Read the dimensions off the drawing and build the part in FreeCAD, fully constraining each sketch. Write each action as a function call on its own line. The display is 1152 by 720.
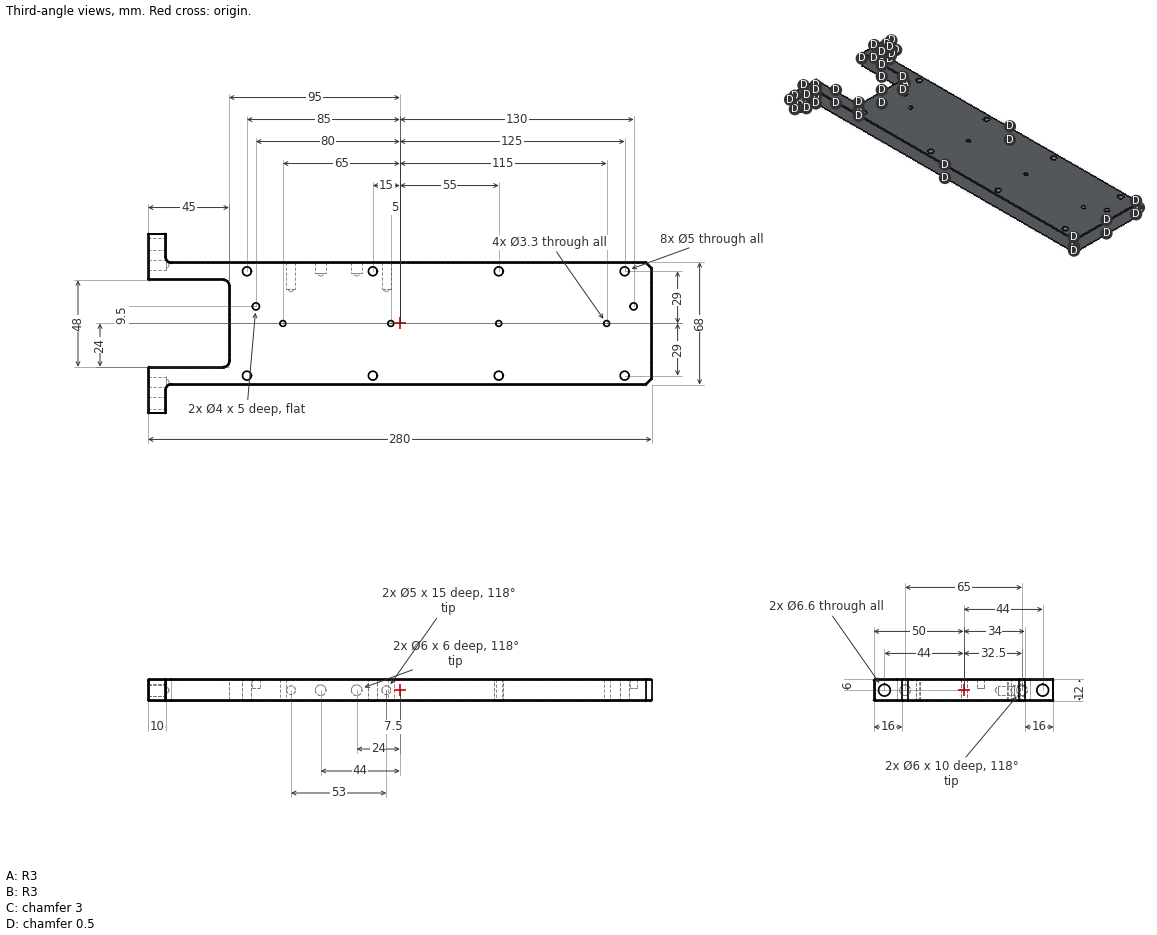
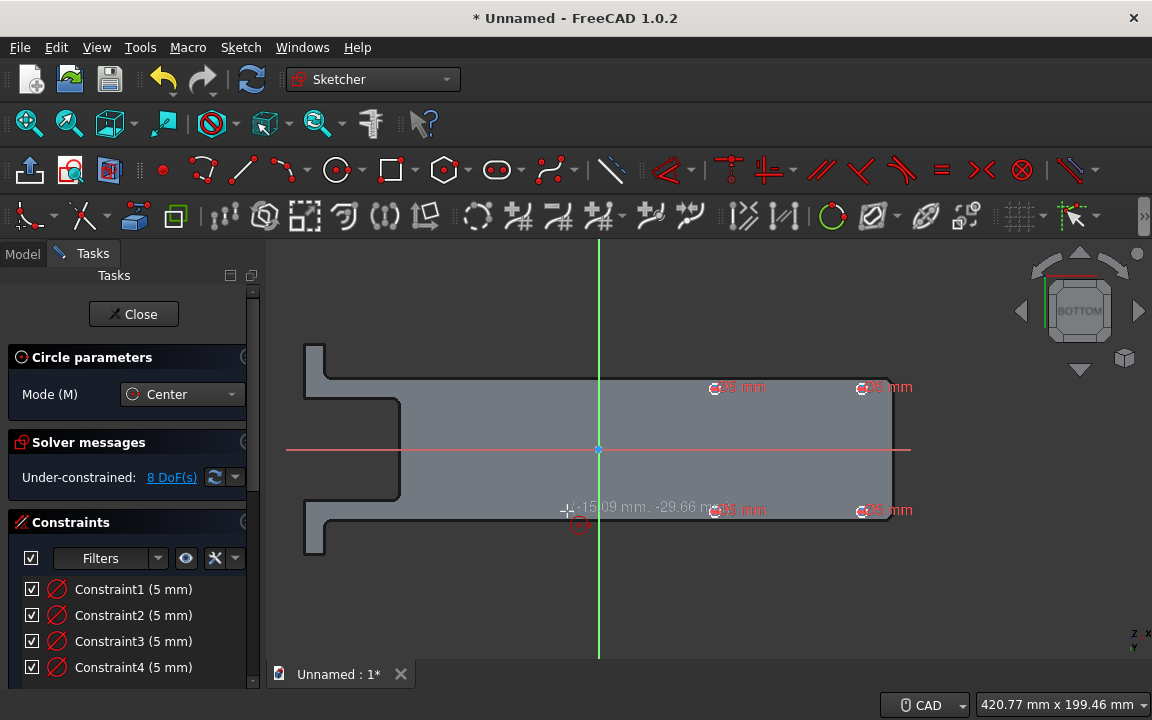
click(567, 511)
move(571, 507)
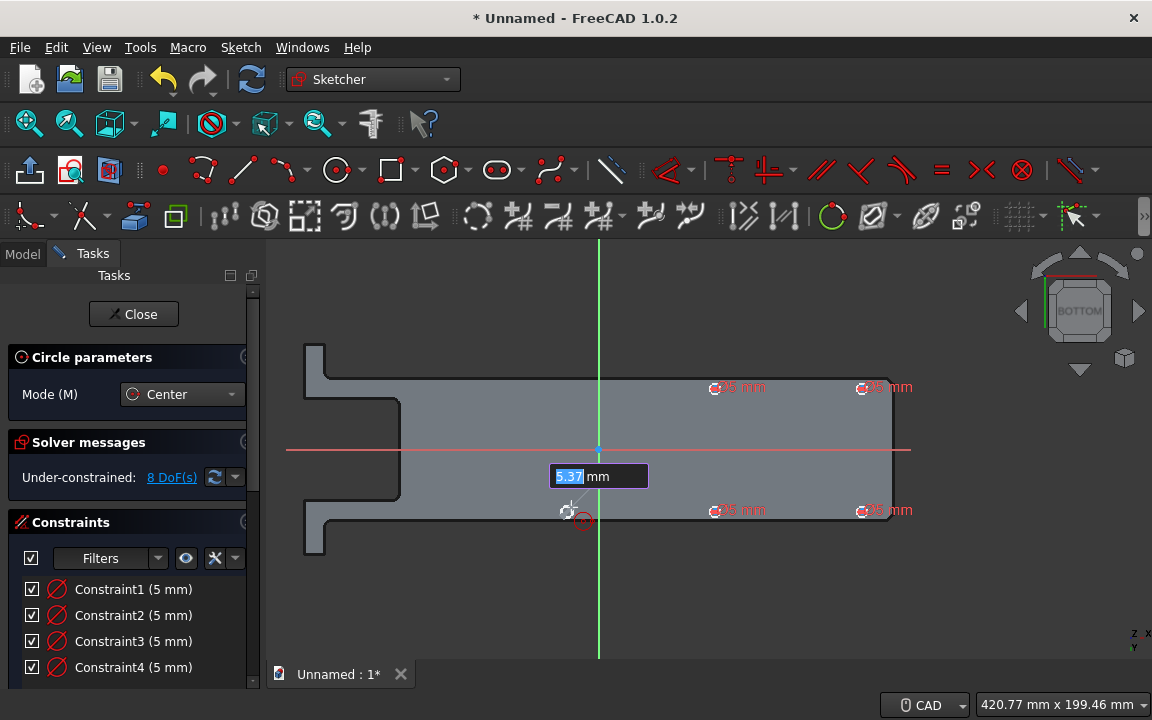
text(5)
key(Return)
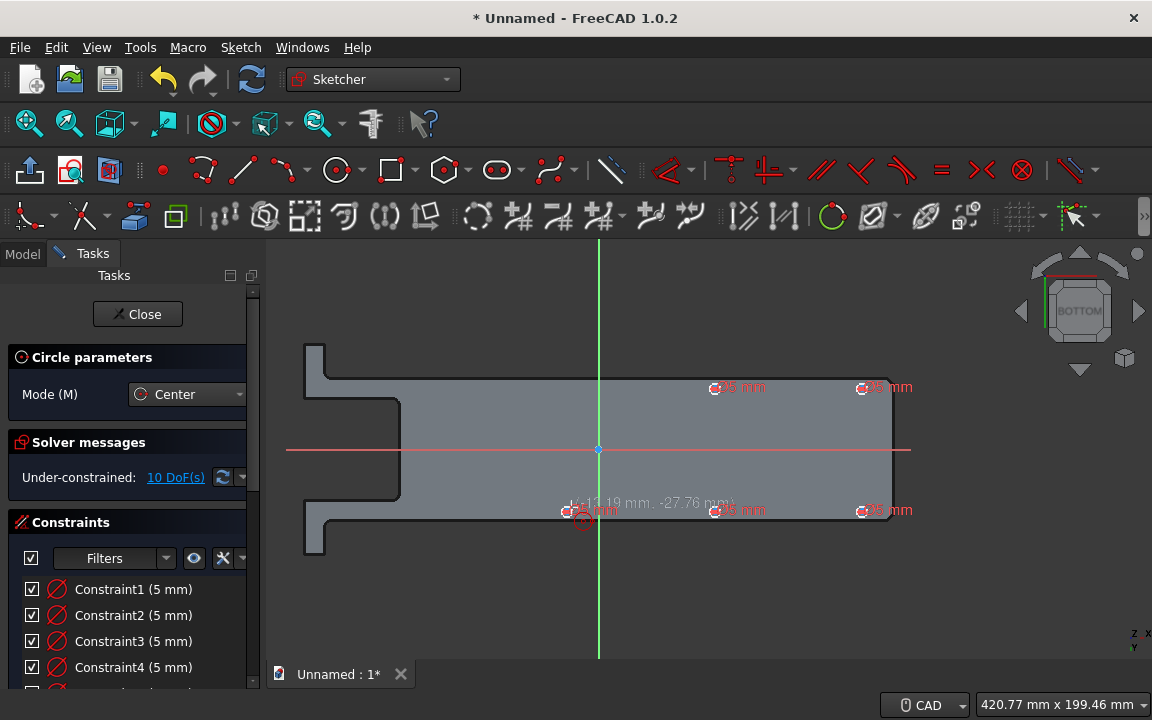
scroll(567, 388, up, 8)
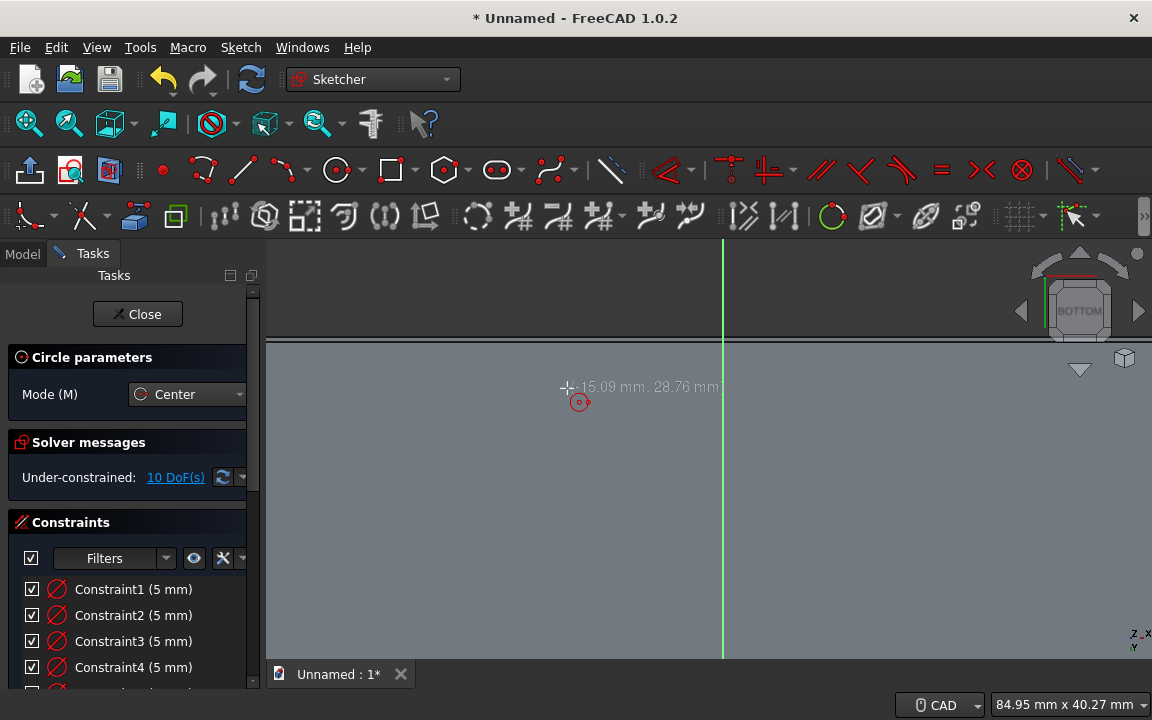
scroll(567, 388, down, 8)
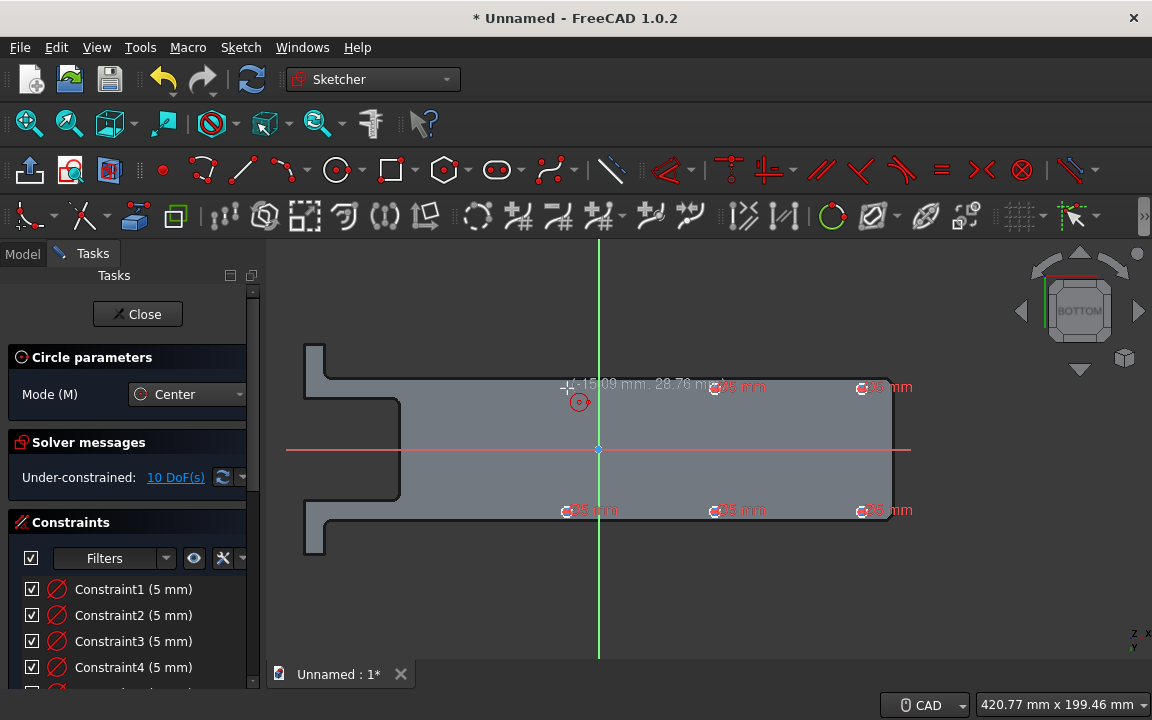
click(567, 388)
move(571, 385)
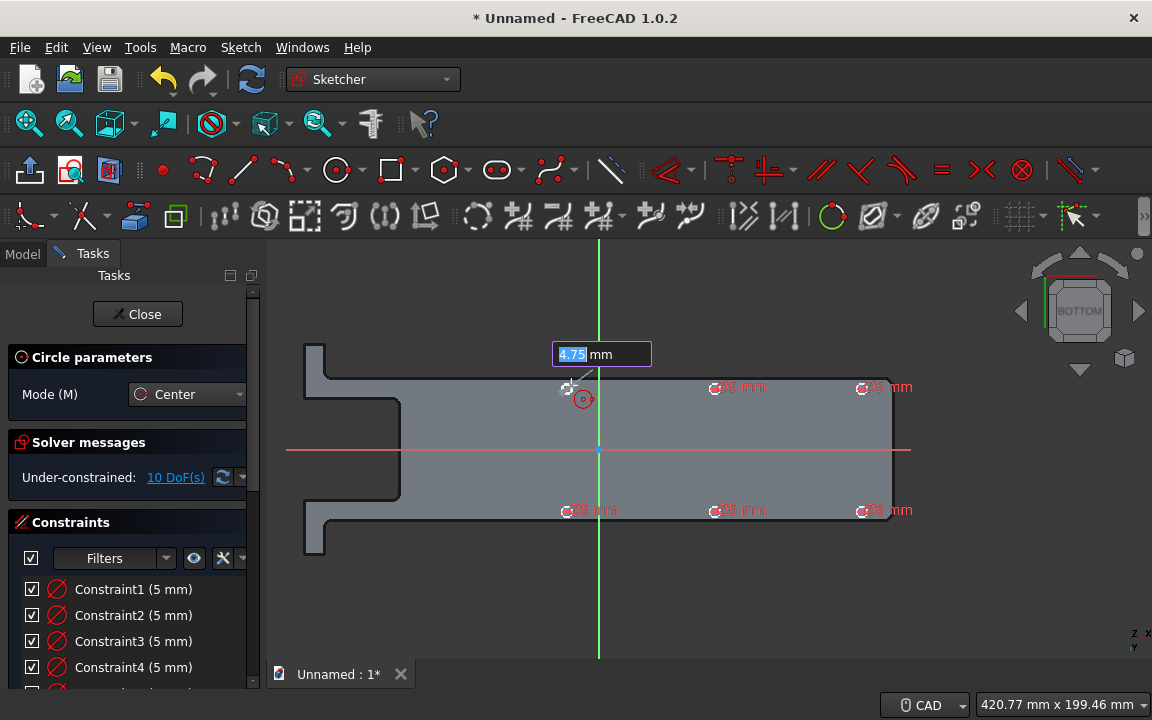
text(5)
key(Return)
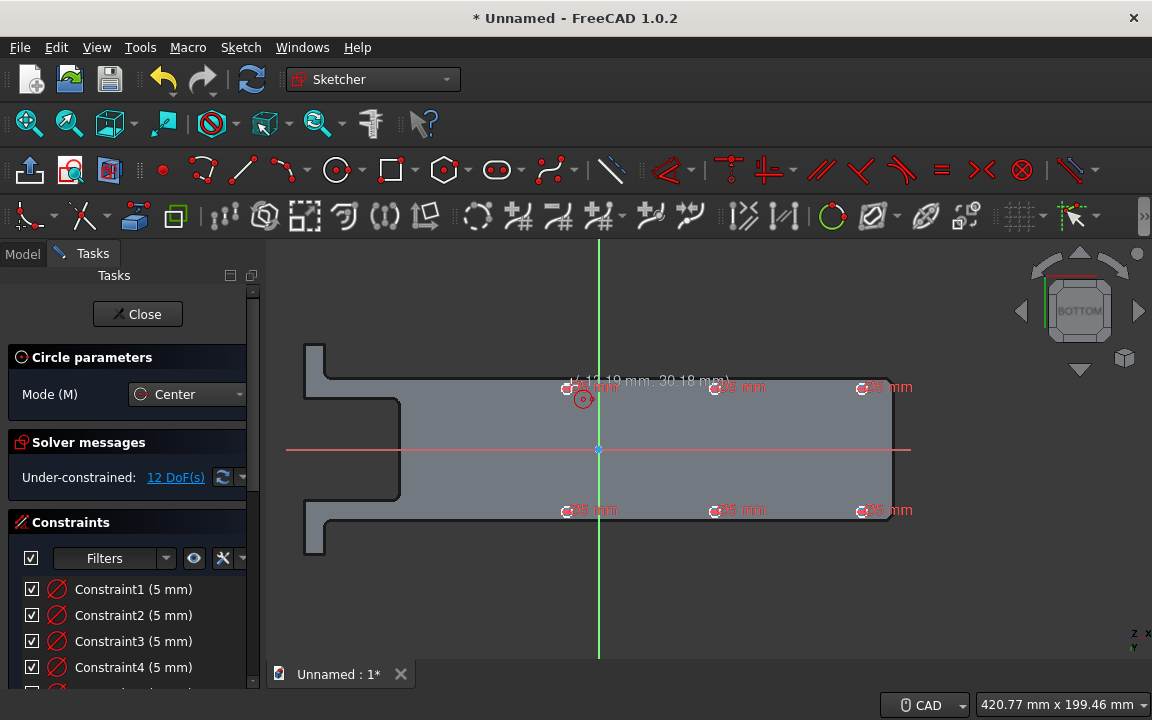
scroll(420, 511, up, 8)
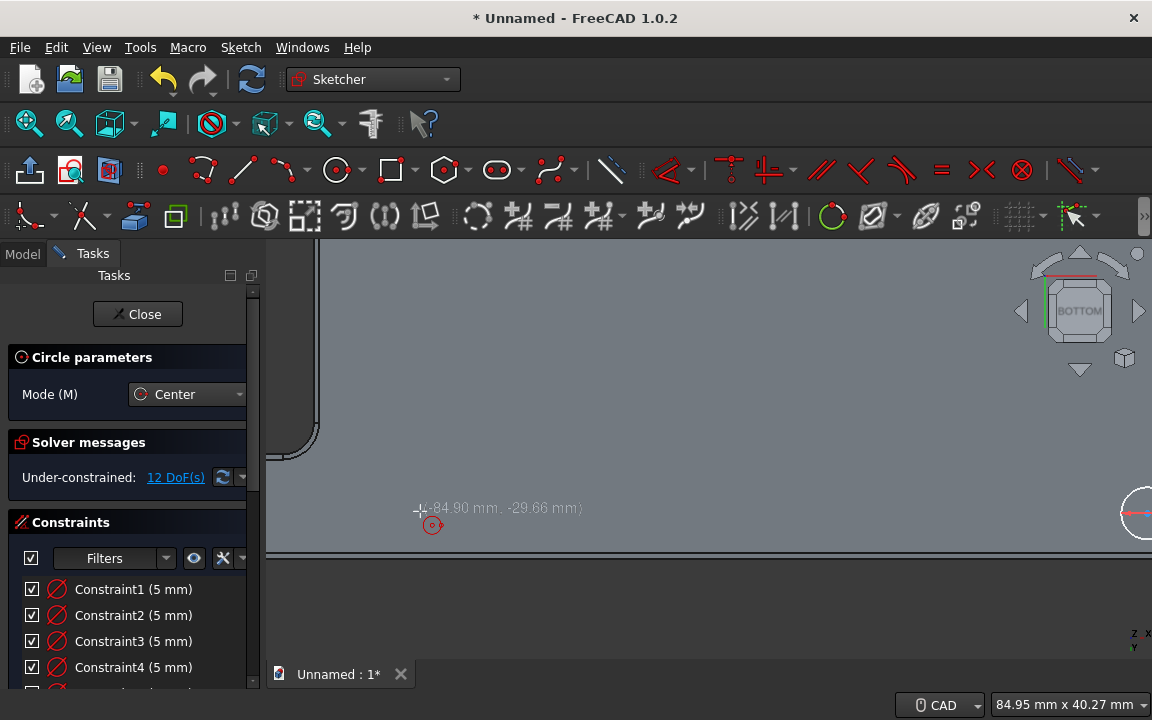
scroll(420, 511, down, 8)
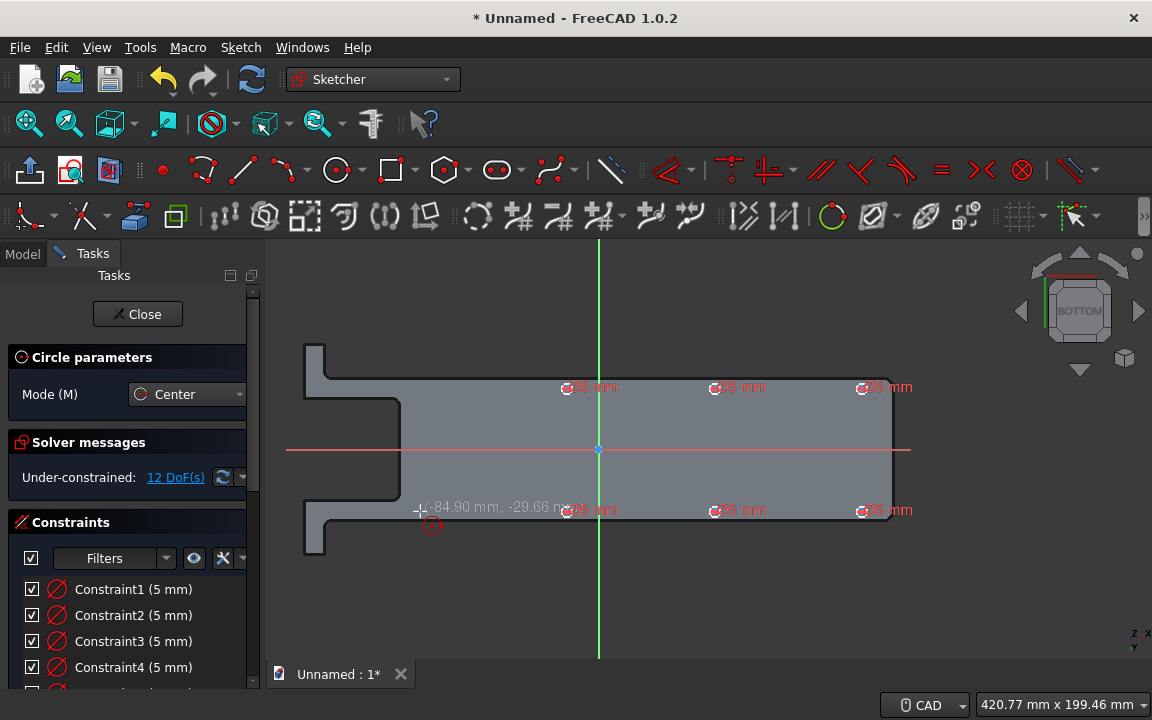
click(420, 511)
move(424, 507)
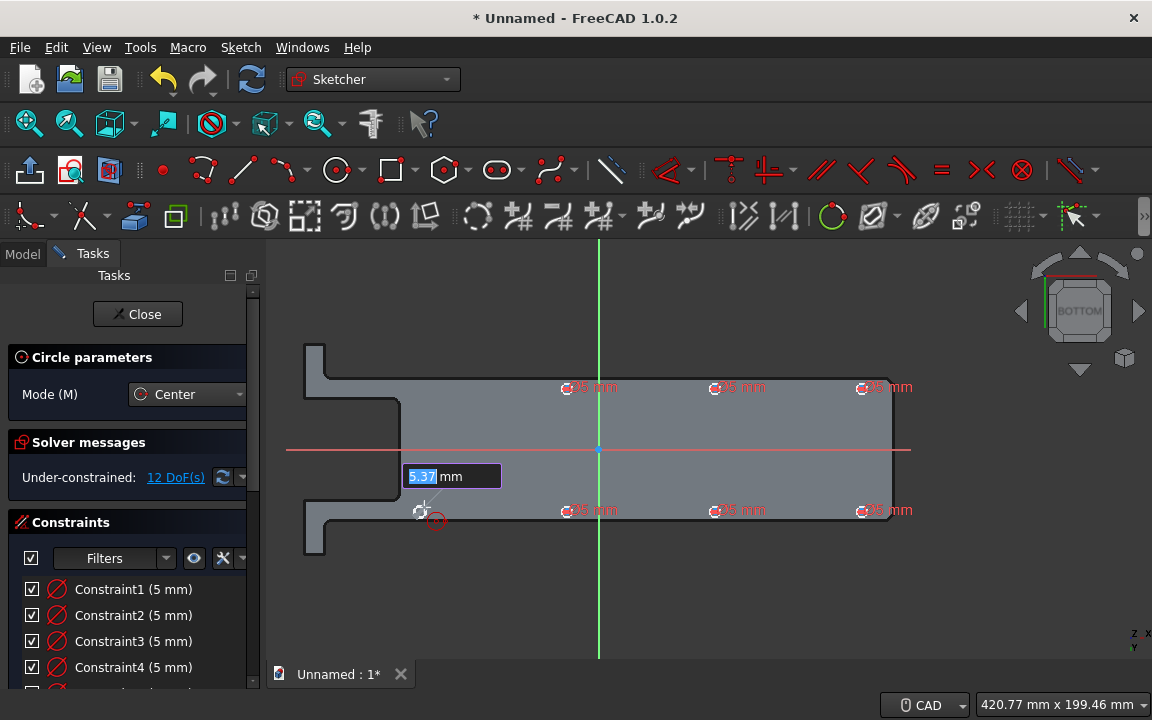
text(5)
key(Return)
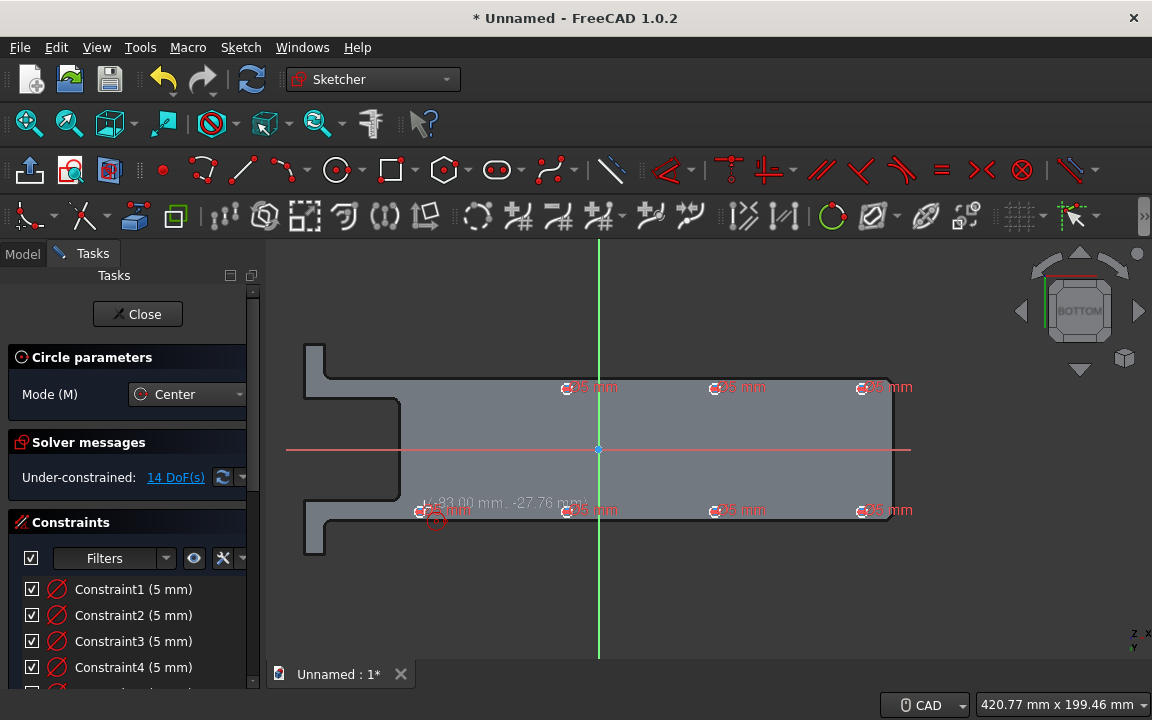
scroll(420, 388, up, 8)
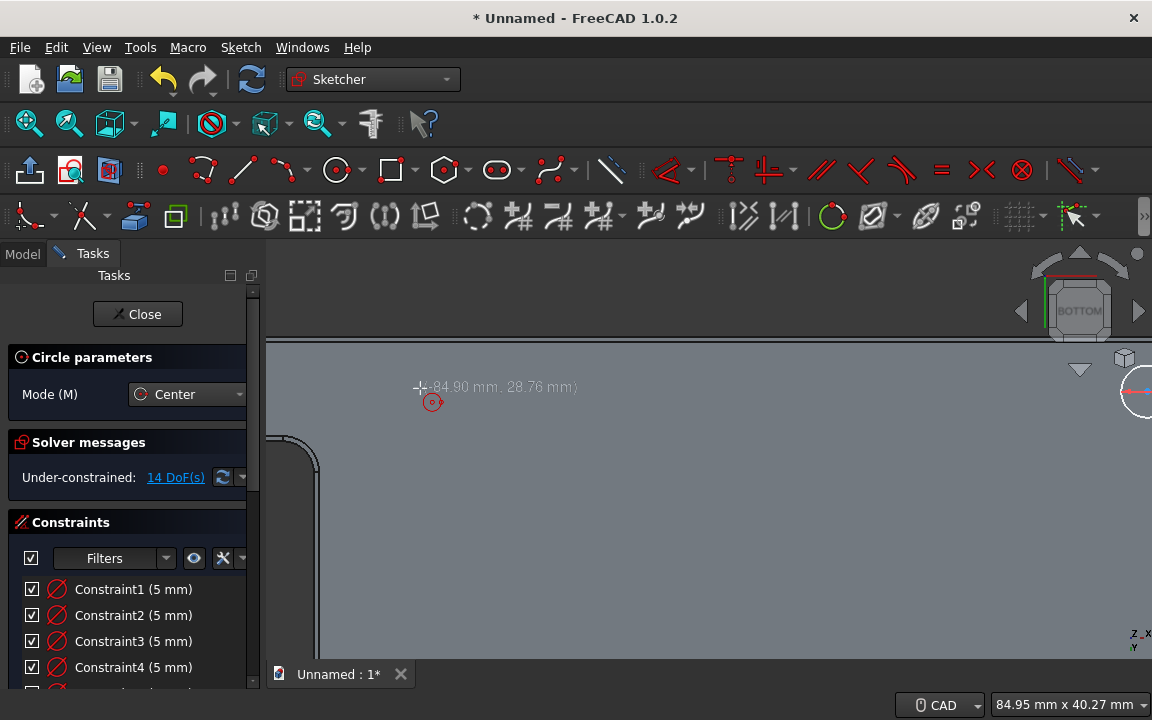
scroll(420, 388, down, 8)